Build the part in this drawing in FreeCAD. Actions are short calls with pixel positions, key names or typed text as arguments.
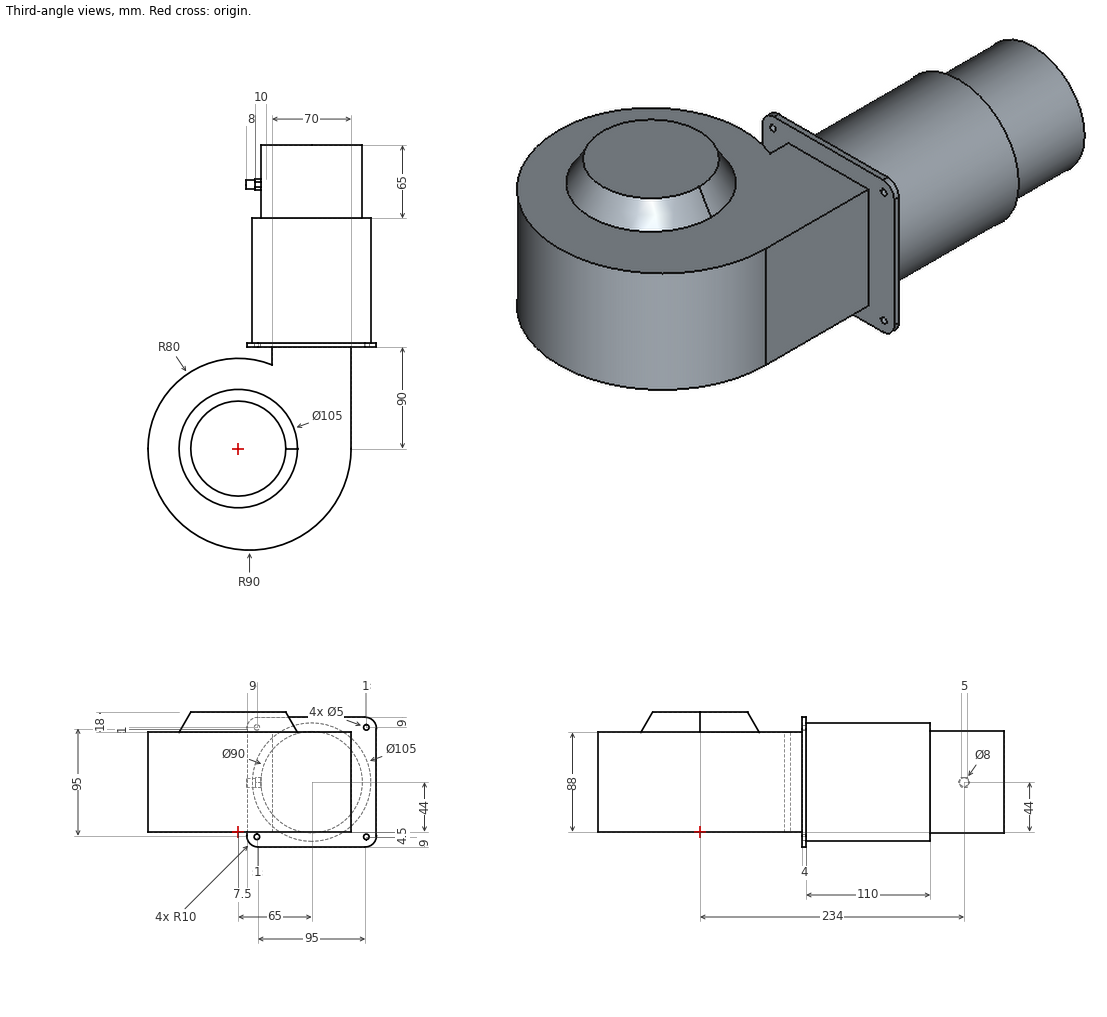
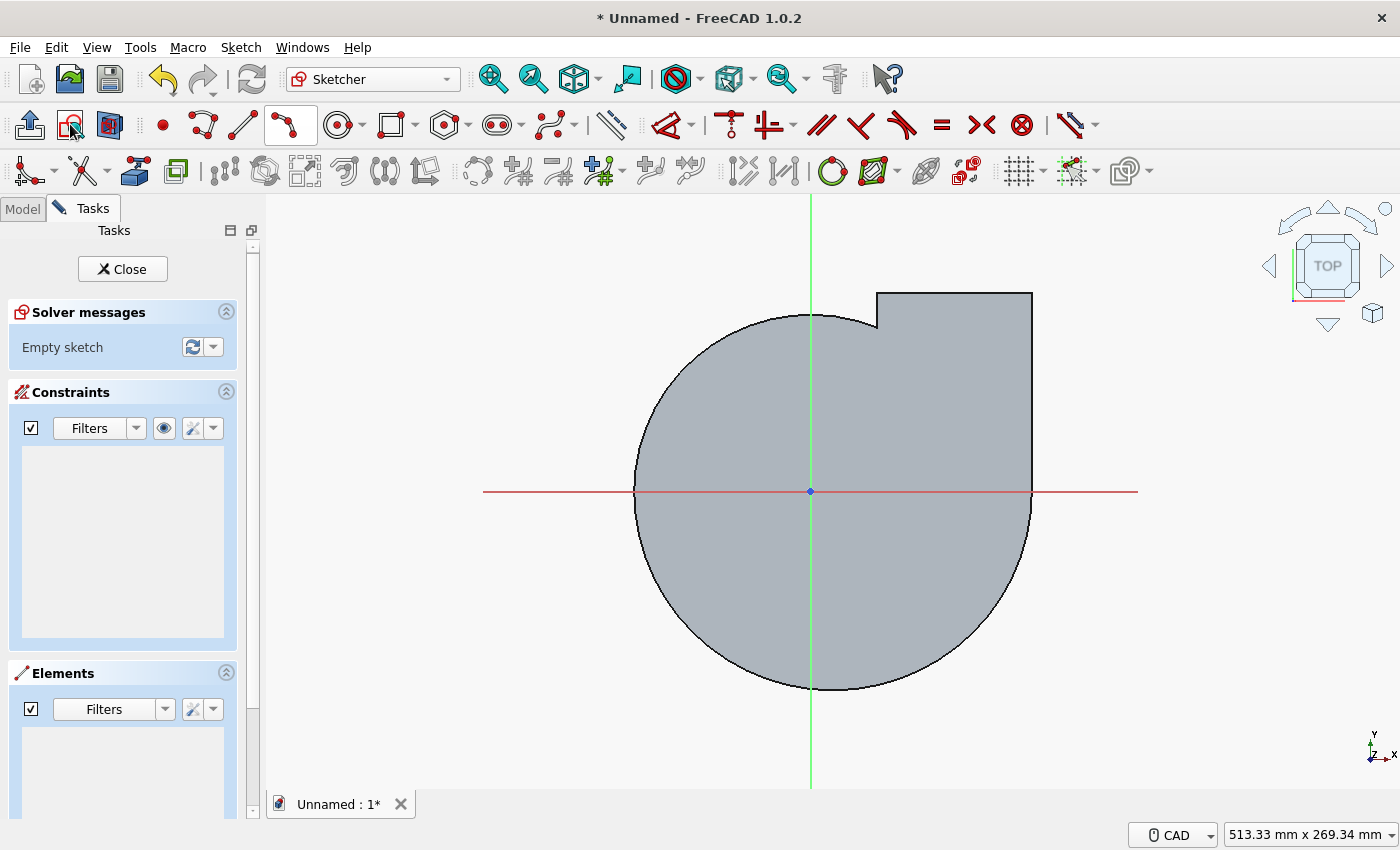
scroll(905, 491, up, 2)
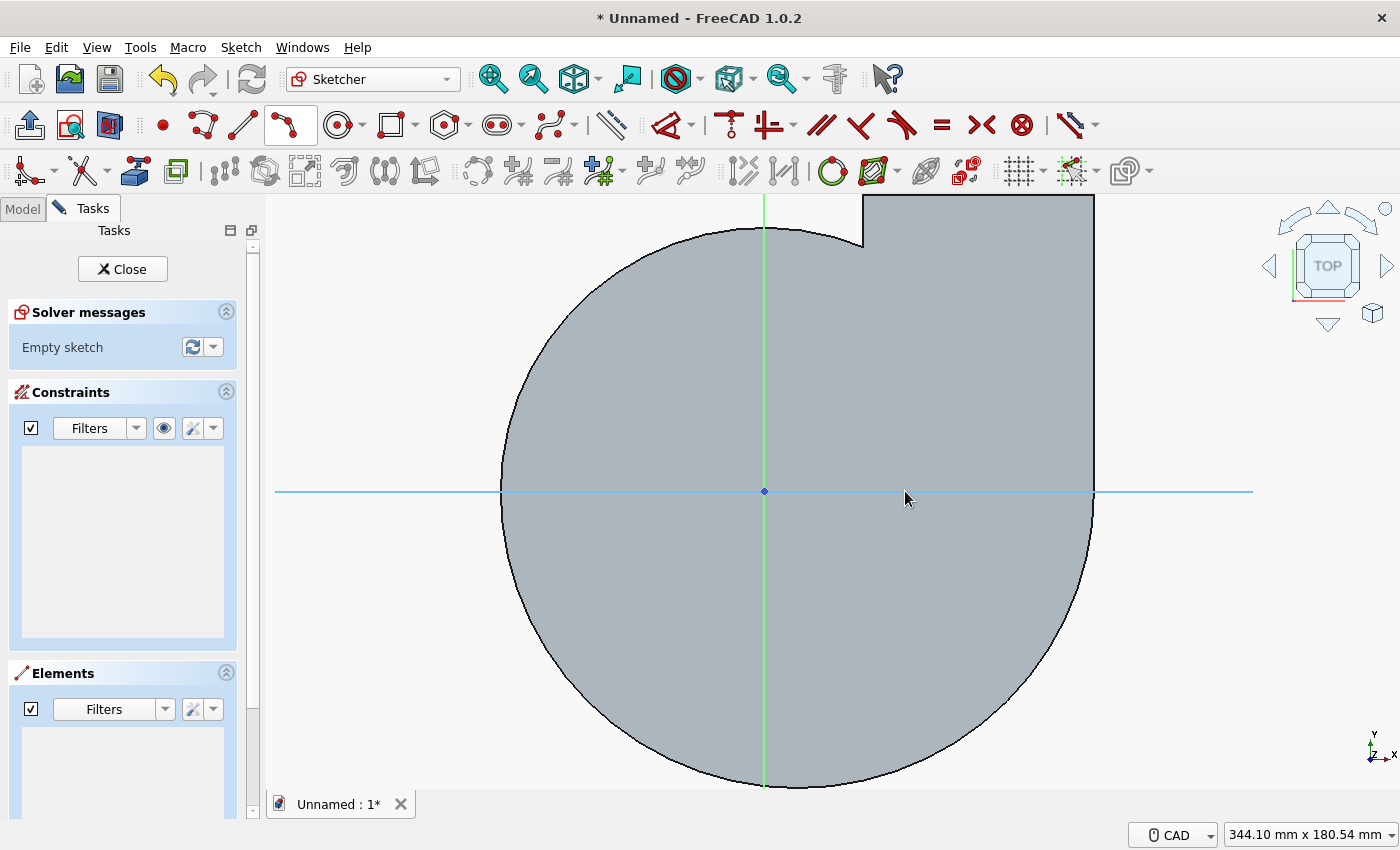
click(338, 126)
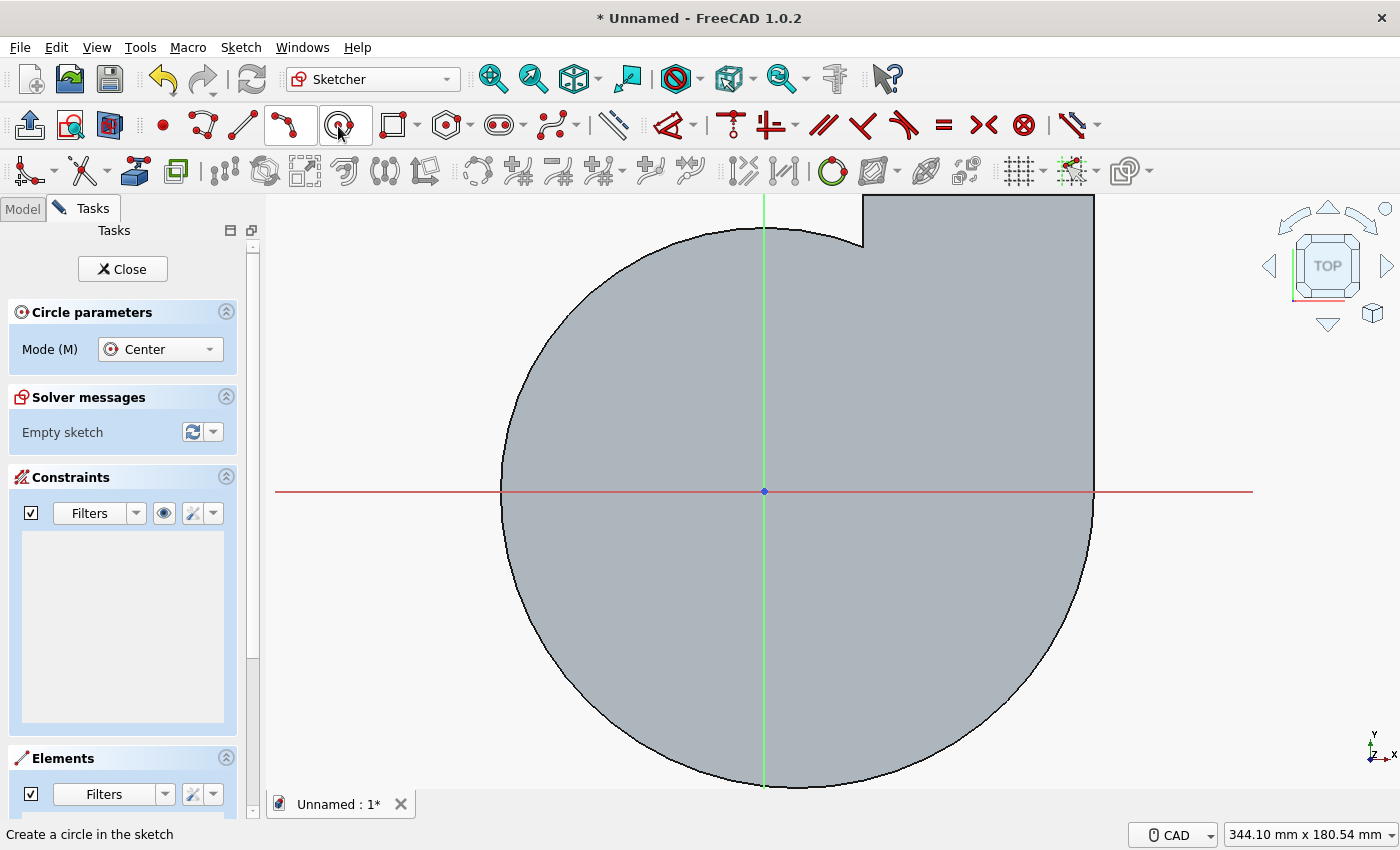
click(764, 492)
click(887, 369)
key(Escape)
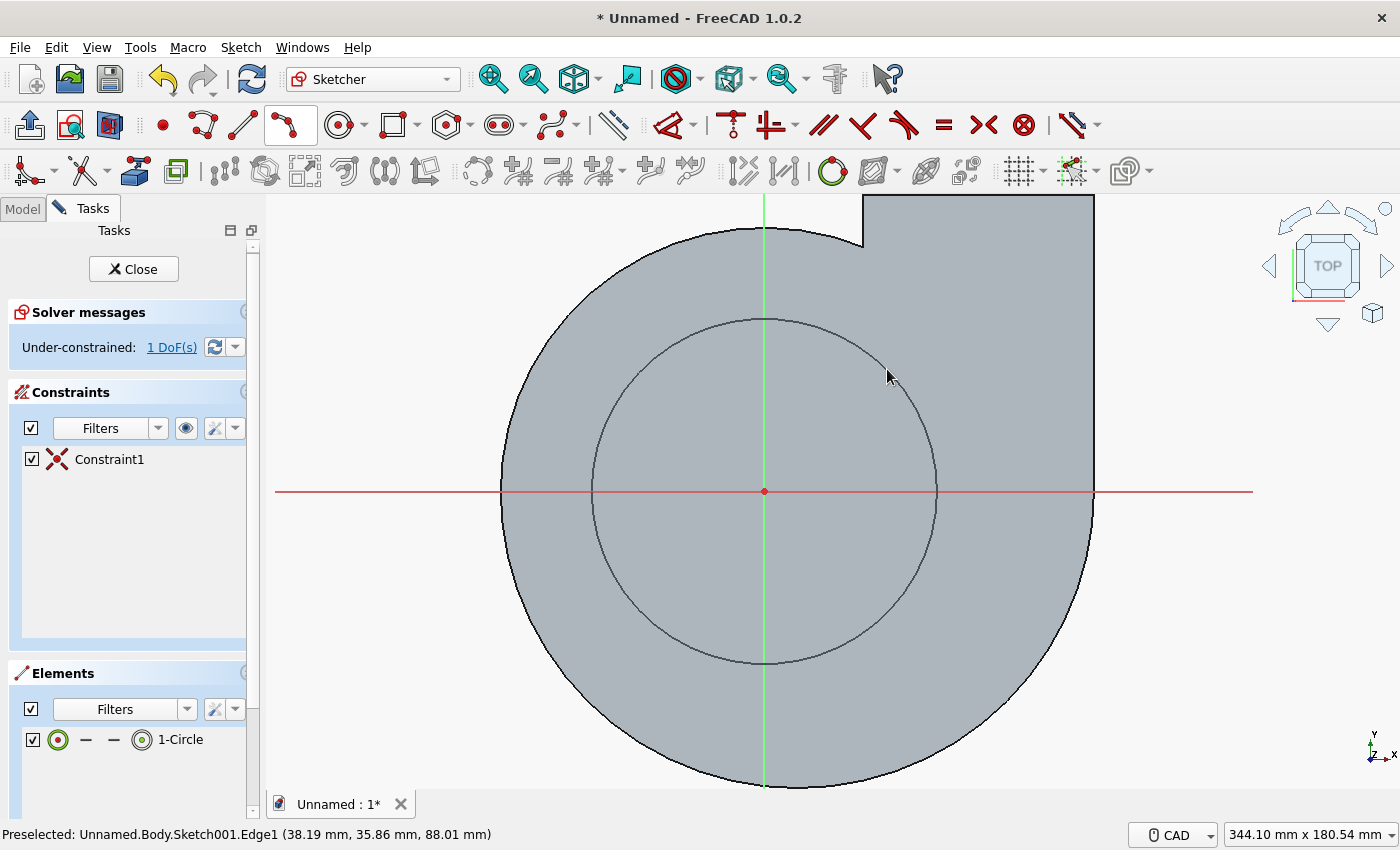
click(668, 126)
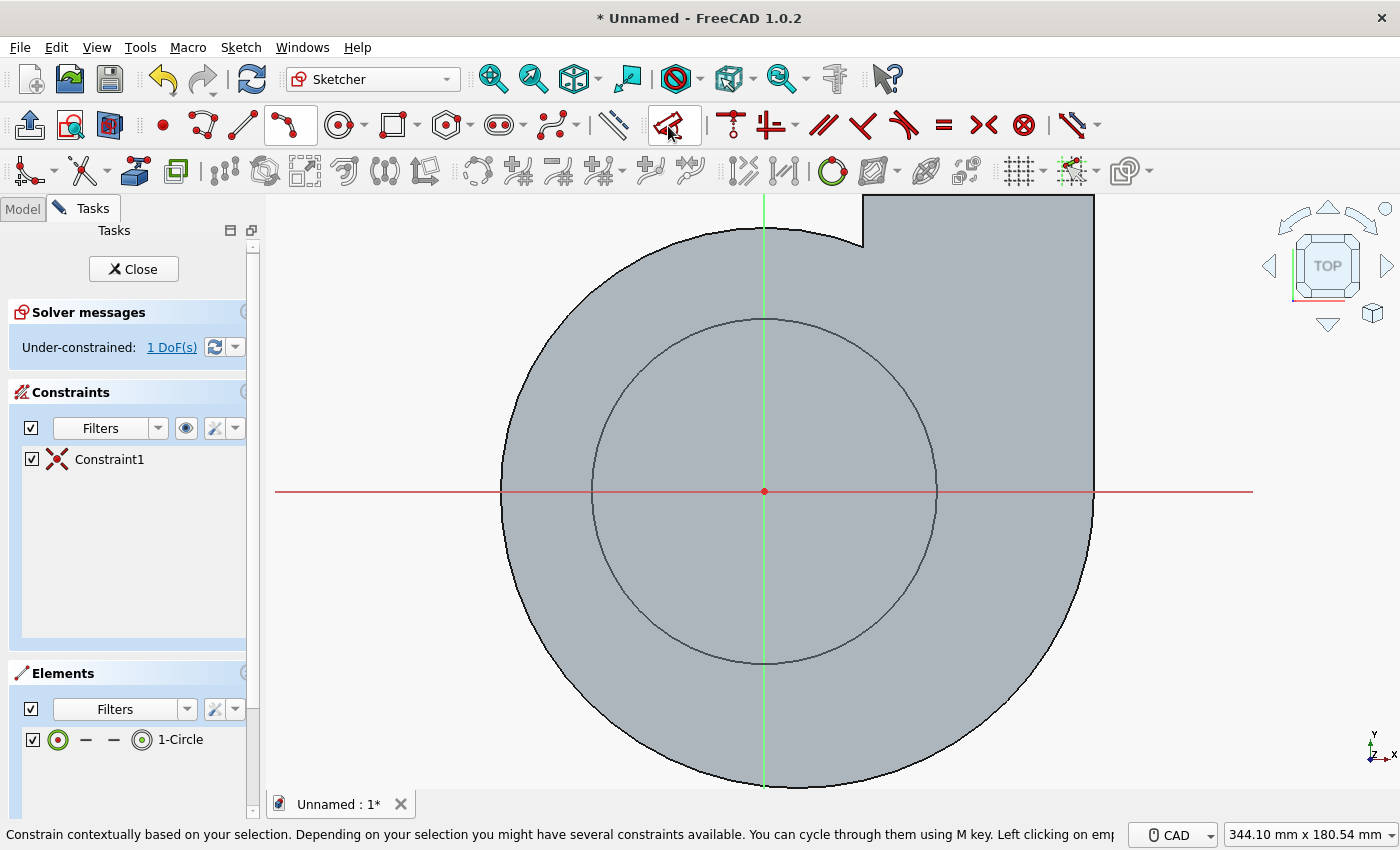
click(886, 369)
click(909, 346)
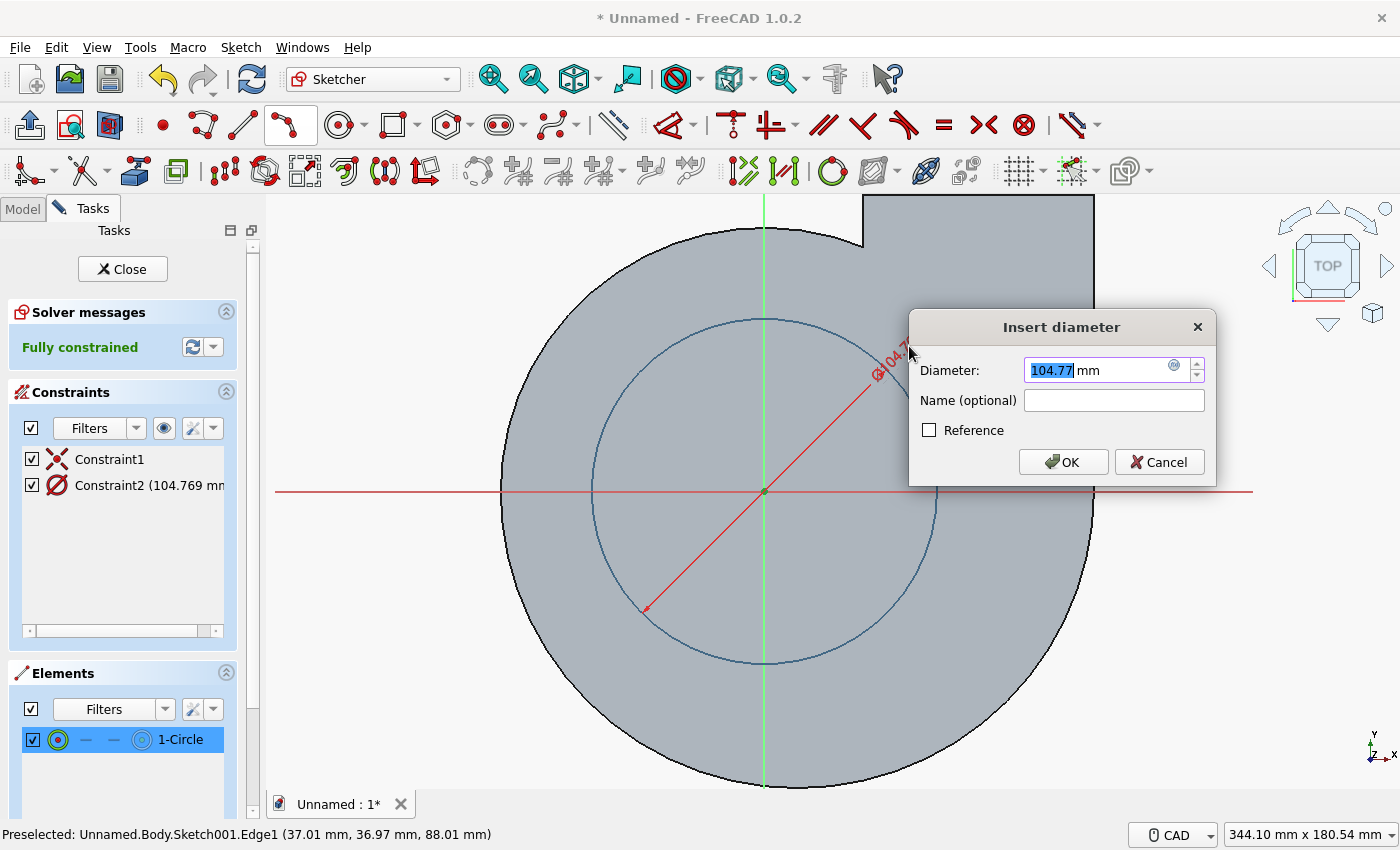
text(105)
key(Return)
key(Escape)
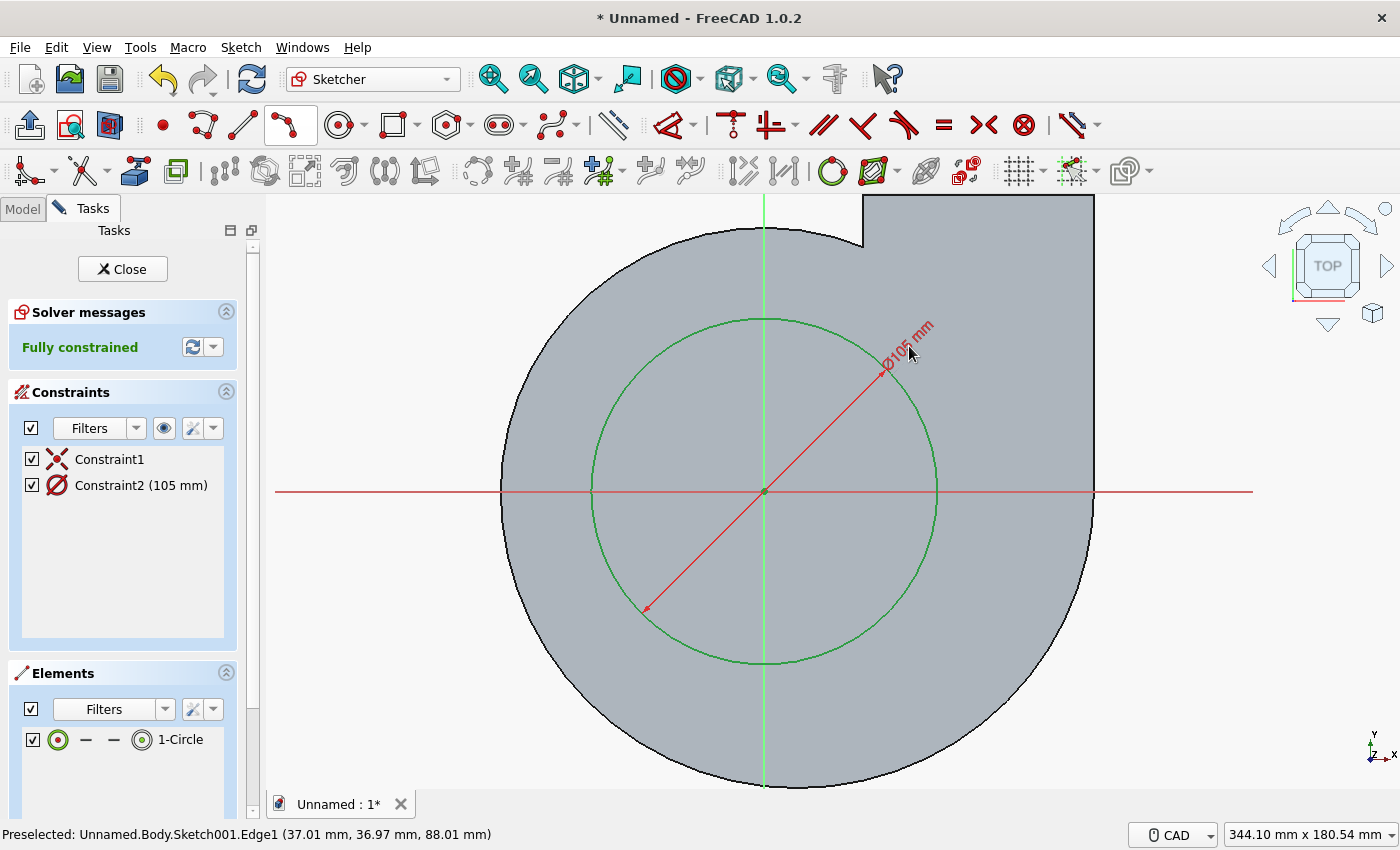
click(123, 269)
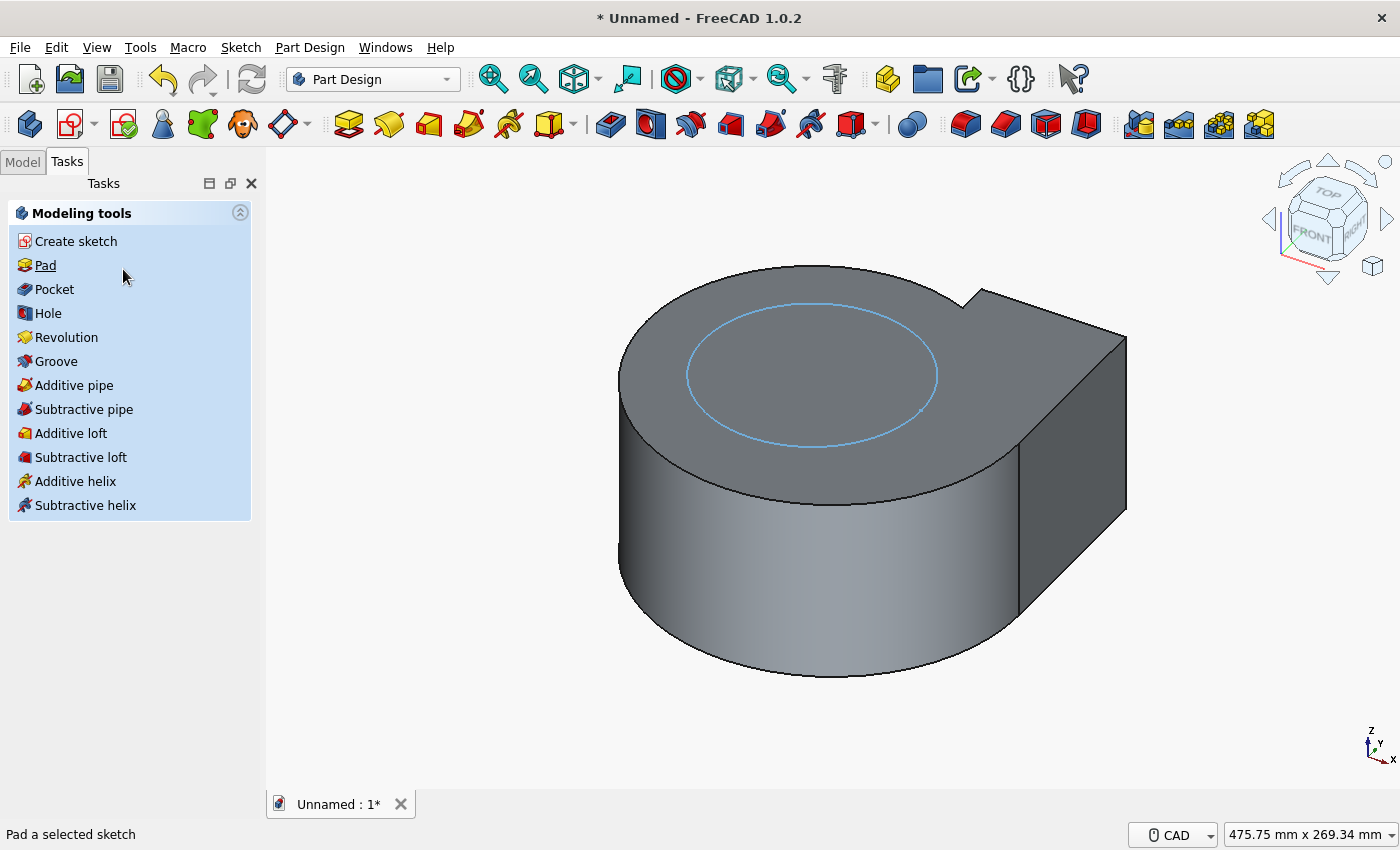
click(350, 124)